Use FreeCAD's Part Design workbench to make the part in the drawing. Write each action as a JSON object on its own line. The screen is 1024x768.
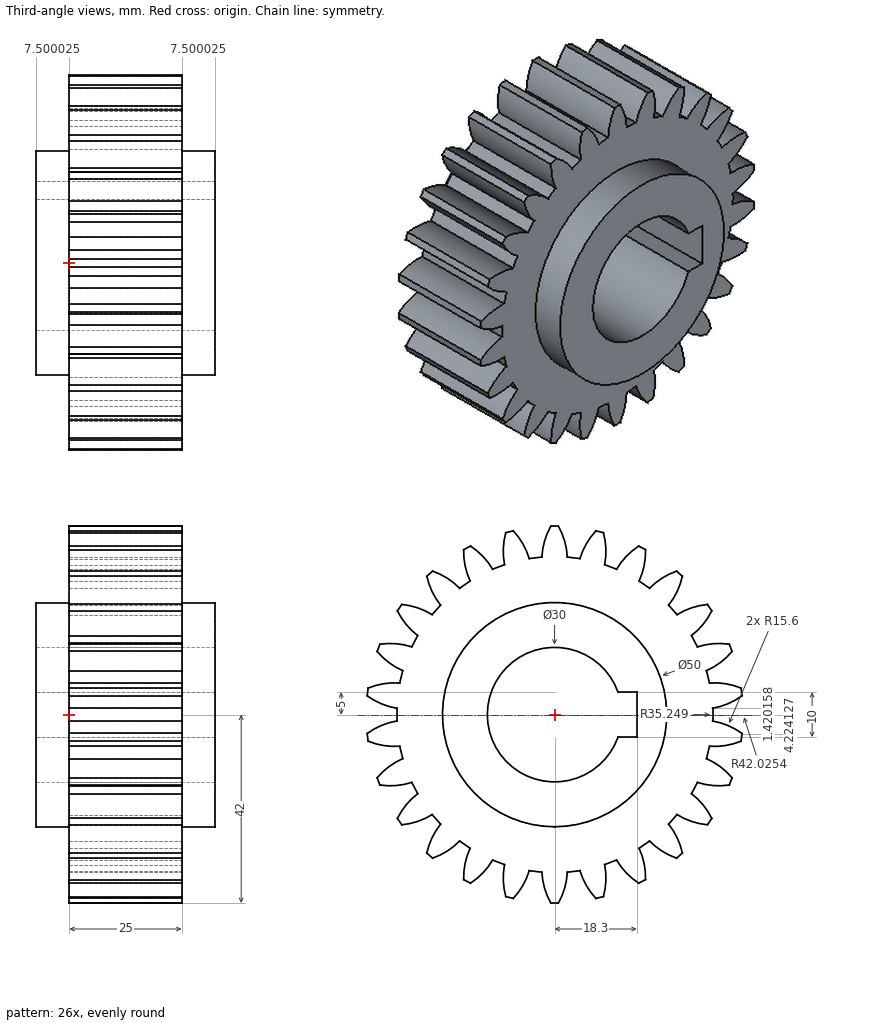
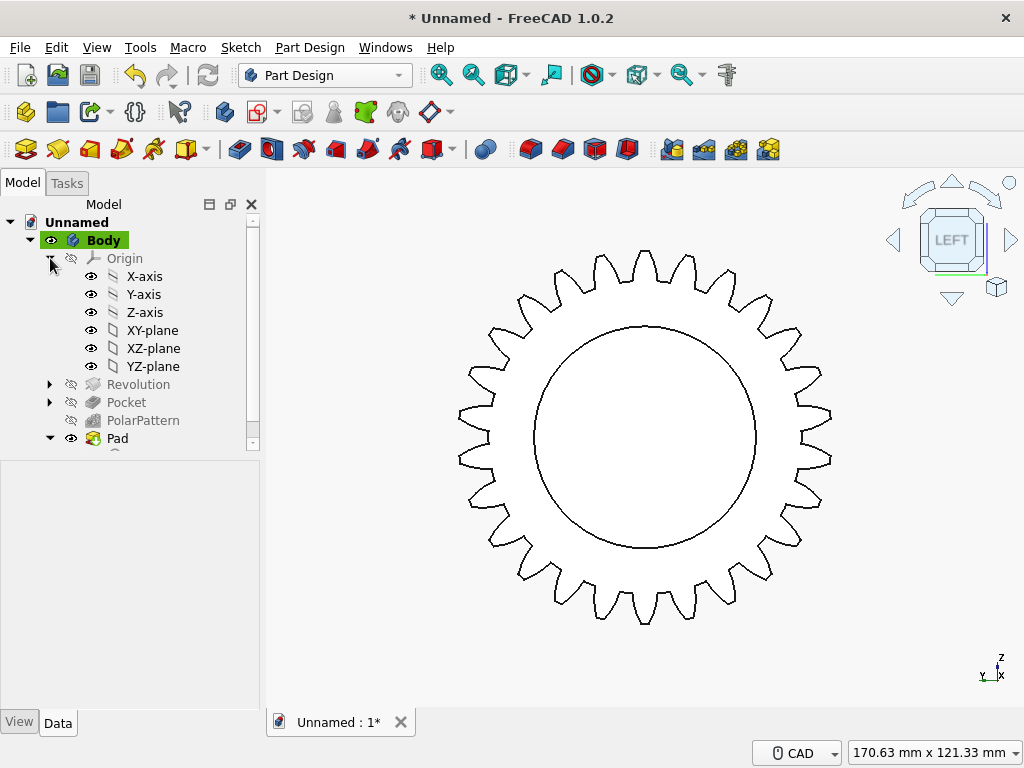
{"action": "left_click", "coordinate": [136, 366]}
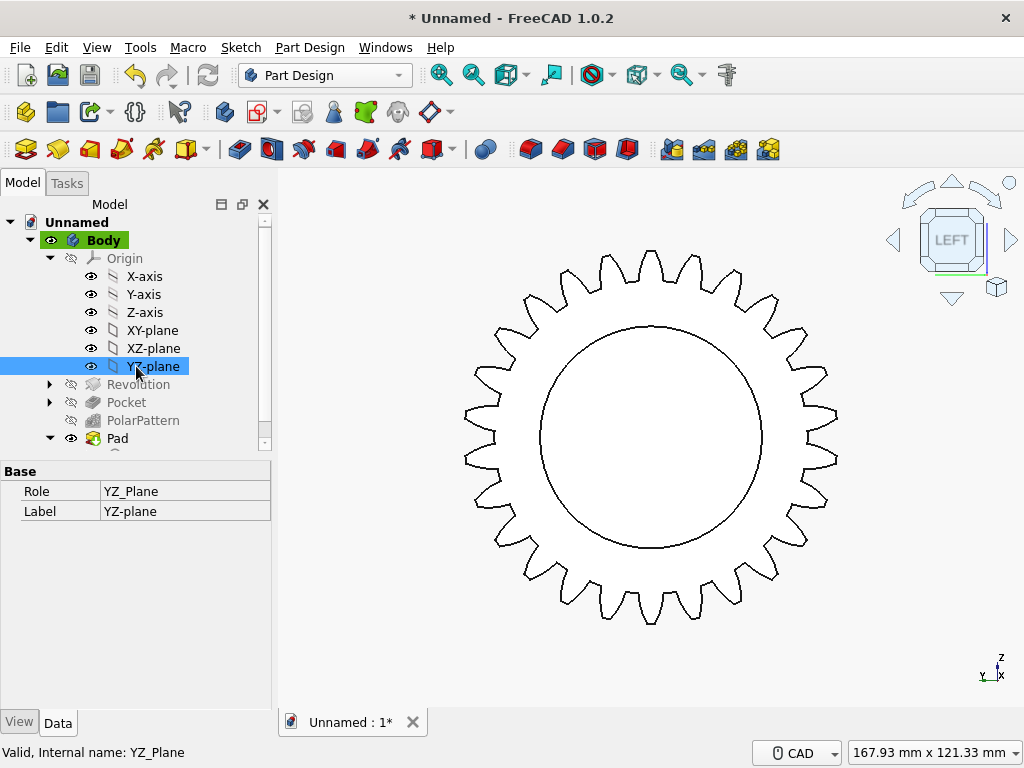
{"action": "left_click", "coordinate": [430, 112]}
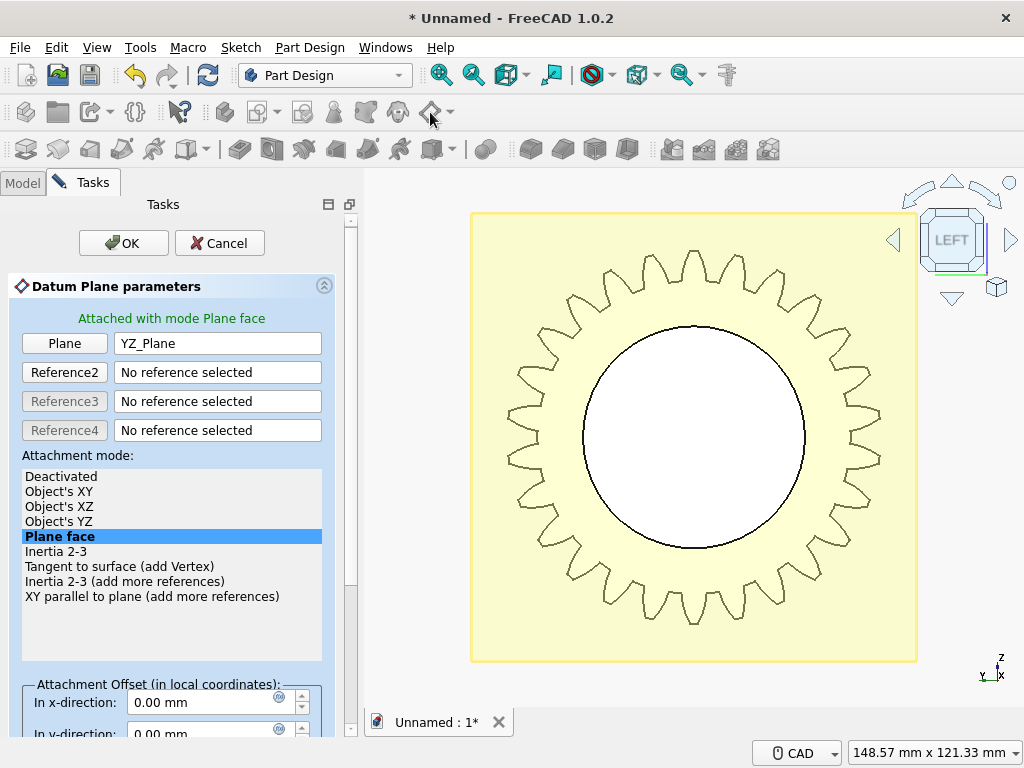
{"action": "scroll", "coordinate": [351, 475], "scroll_direction": "down", "scroll_amount": 2}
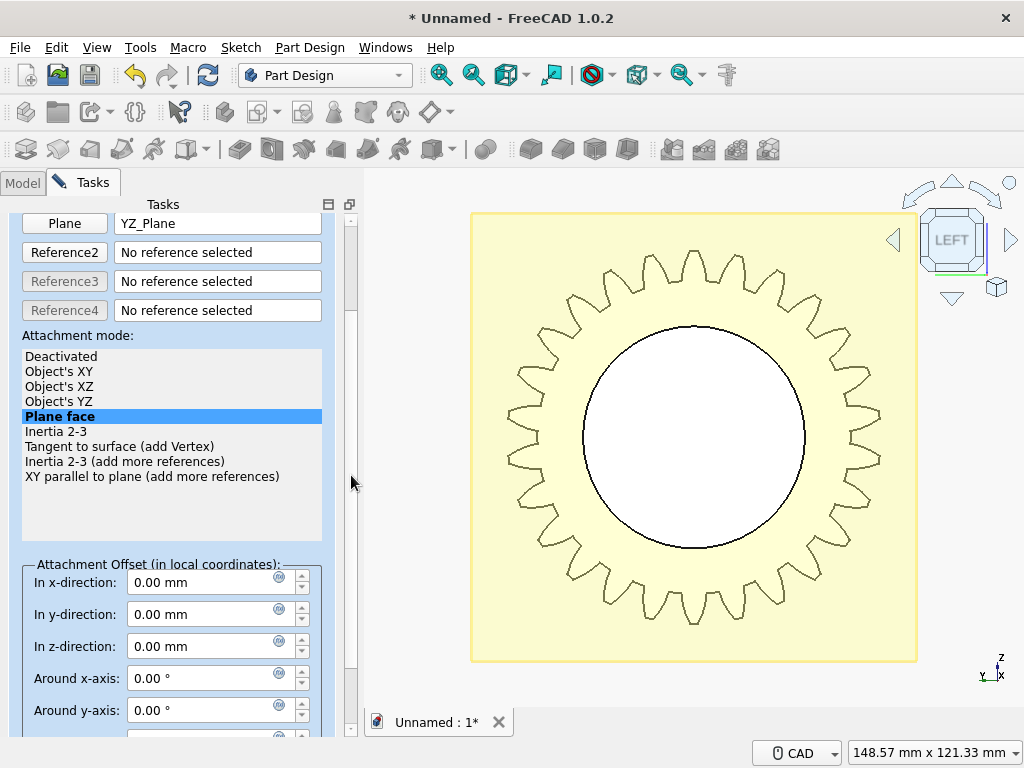
{"action": "triple_click", "coordinate": [210, 646]}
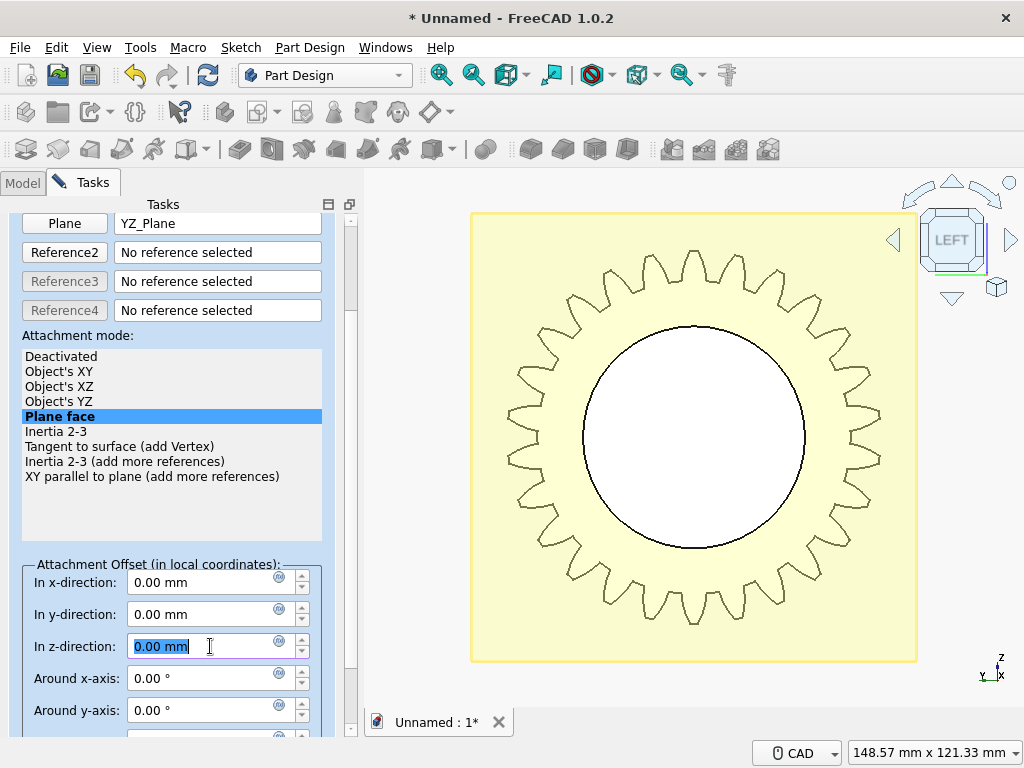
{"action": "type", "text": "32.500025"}
{"action": "key", "text": "Tab"}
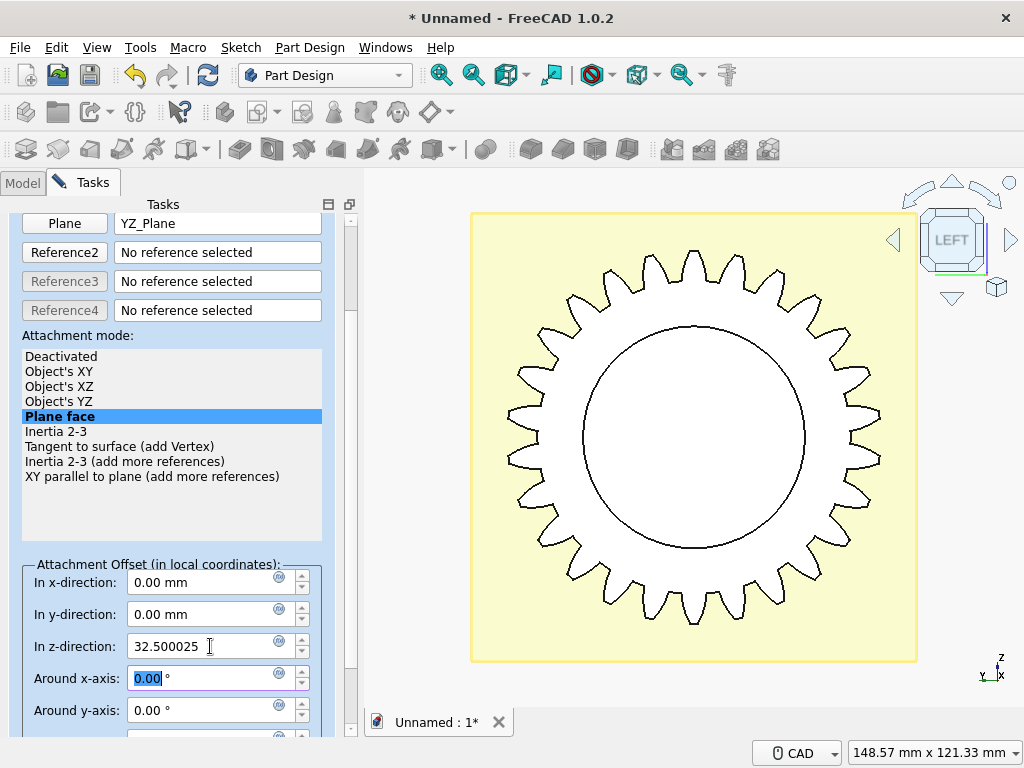
{"action": "scroll", "coordinate": [351, 475], "scroll_direction": "up", "scroll_amount": 3}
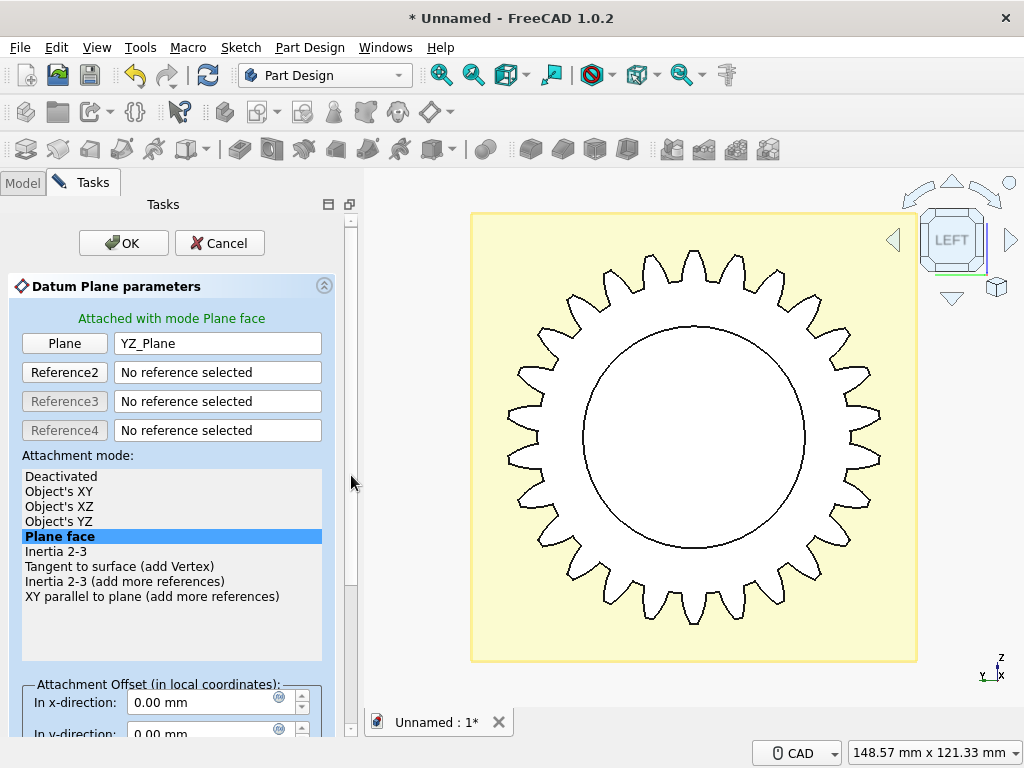
{"action": "left_click", "coordinate": [124, 243]}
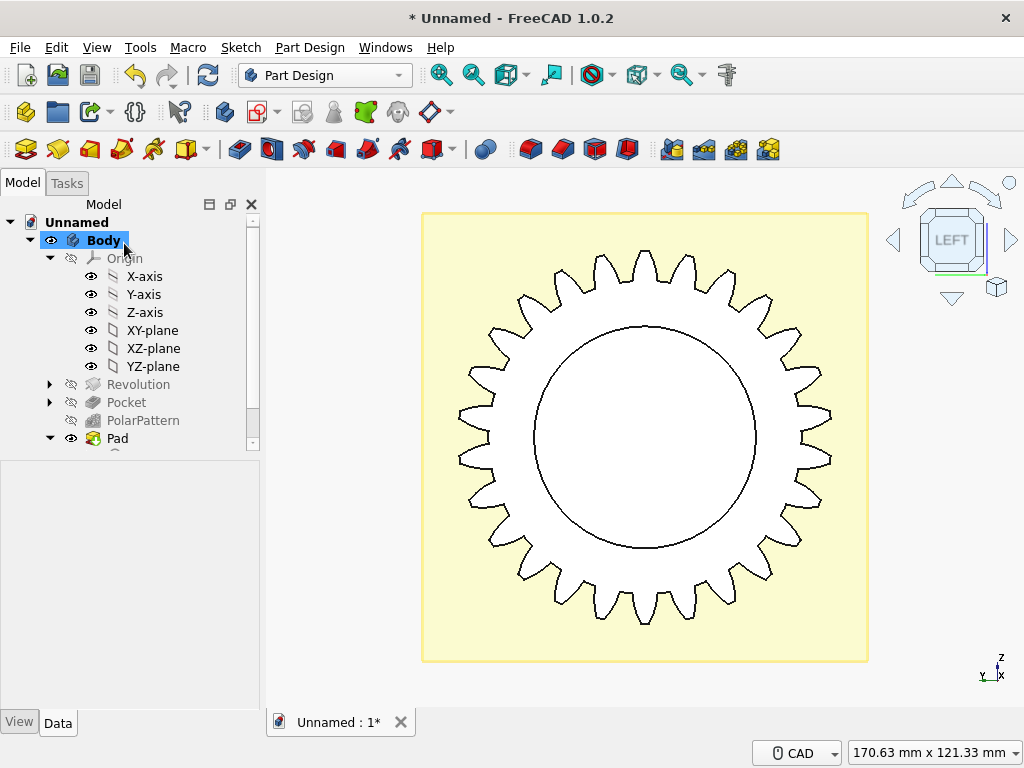
{"action": "scroll", "coordinate": [100, 326], "scroll_direction": "down", "scroll_amount": 3}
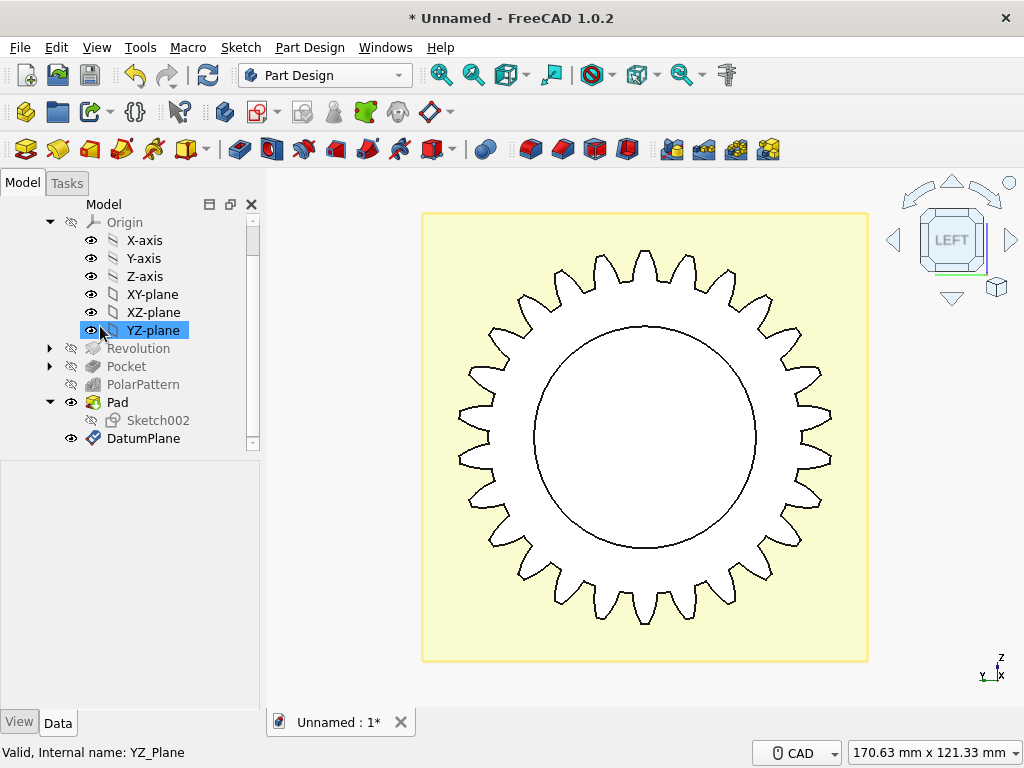
{"action": "left_click", "coordinate": [116, 438]}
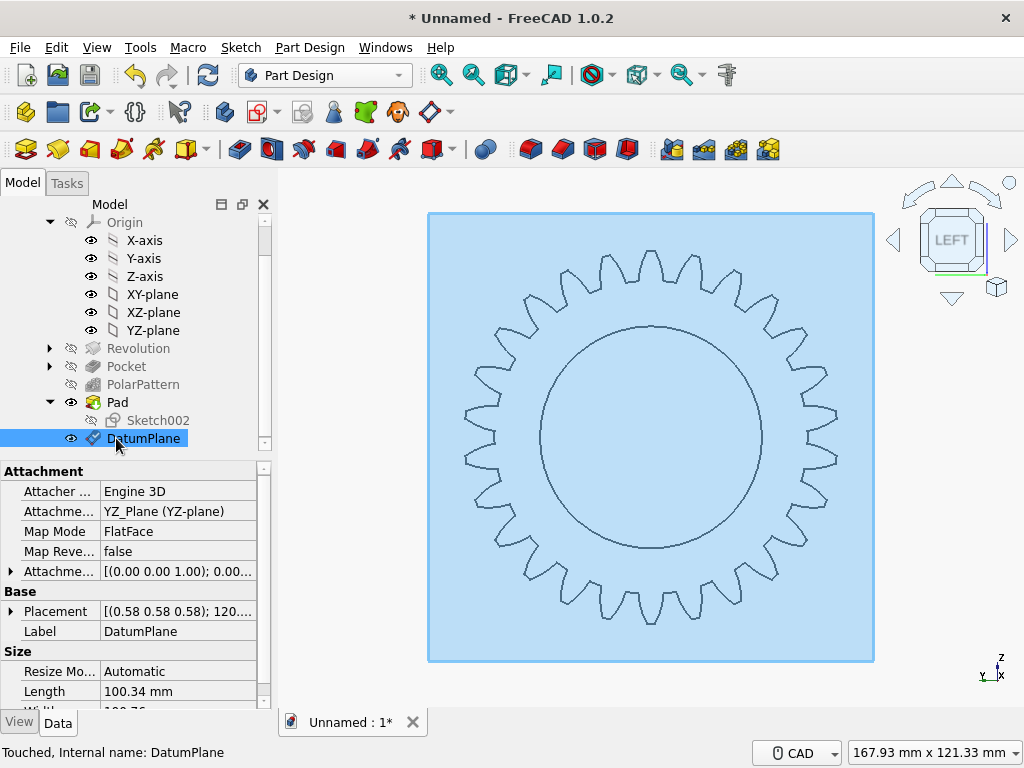
{"action": "left_click", "coordinate": [258, 112]}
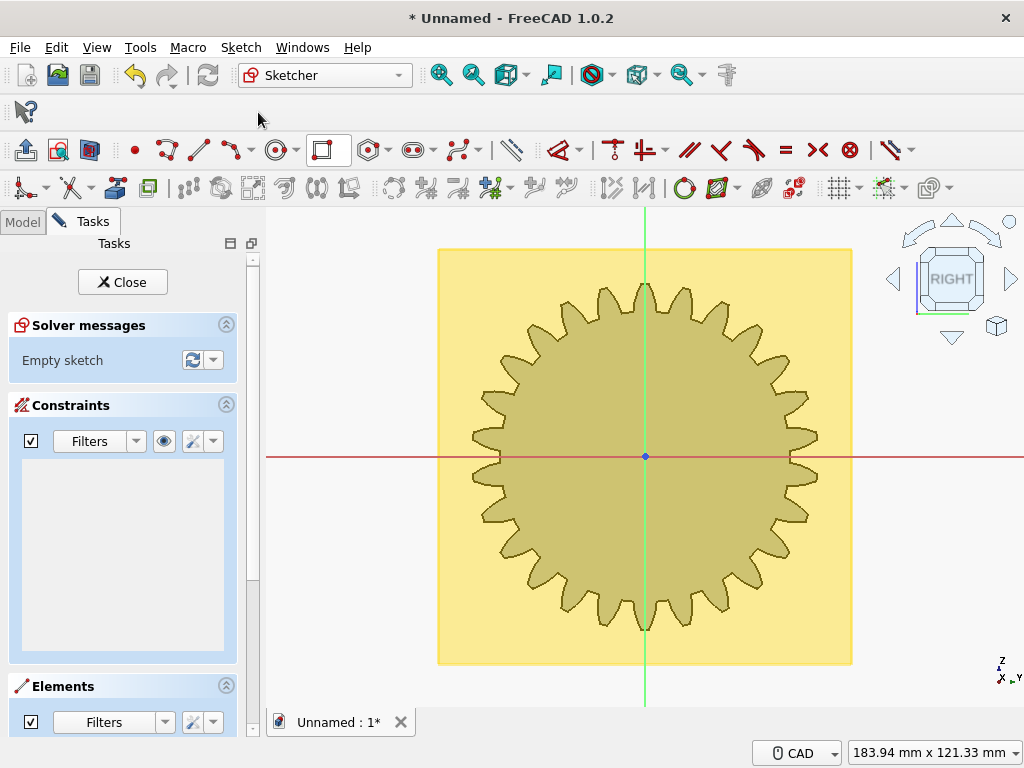
{"action": "scroll", "coordinate": [784, 457], "scroll_direction": "up", "scroll_amount": 2}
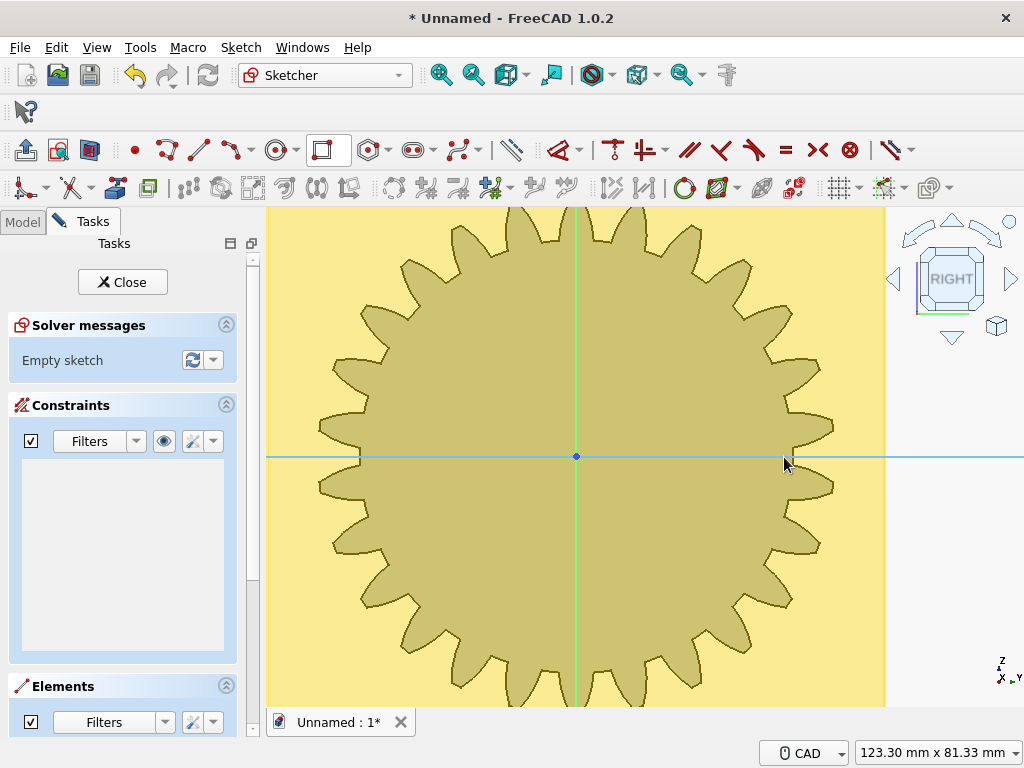
{"action": "left_click", "coordinate": [276, 150]}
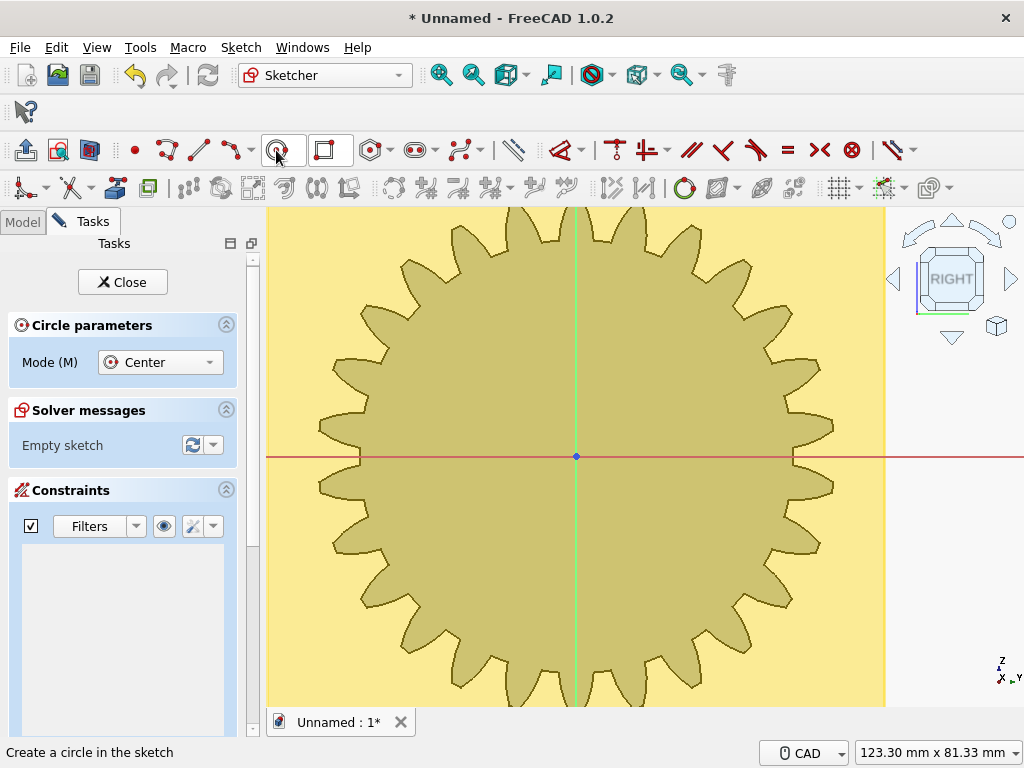
{"action": "left_click", "coordinate": [576, 457]}
{"action": "mouse_move", "coordinate": [685, 348]}